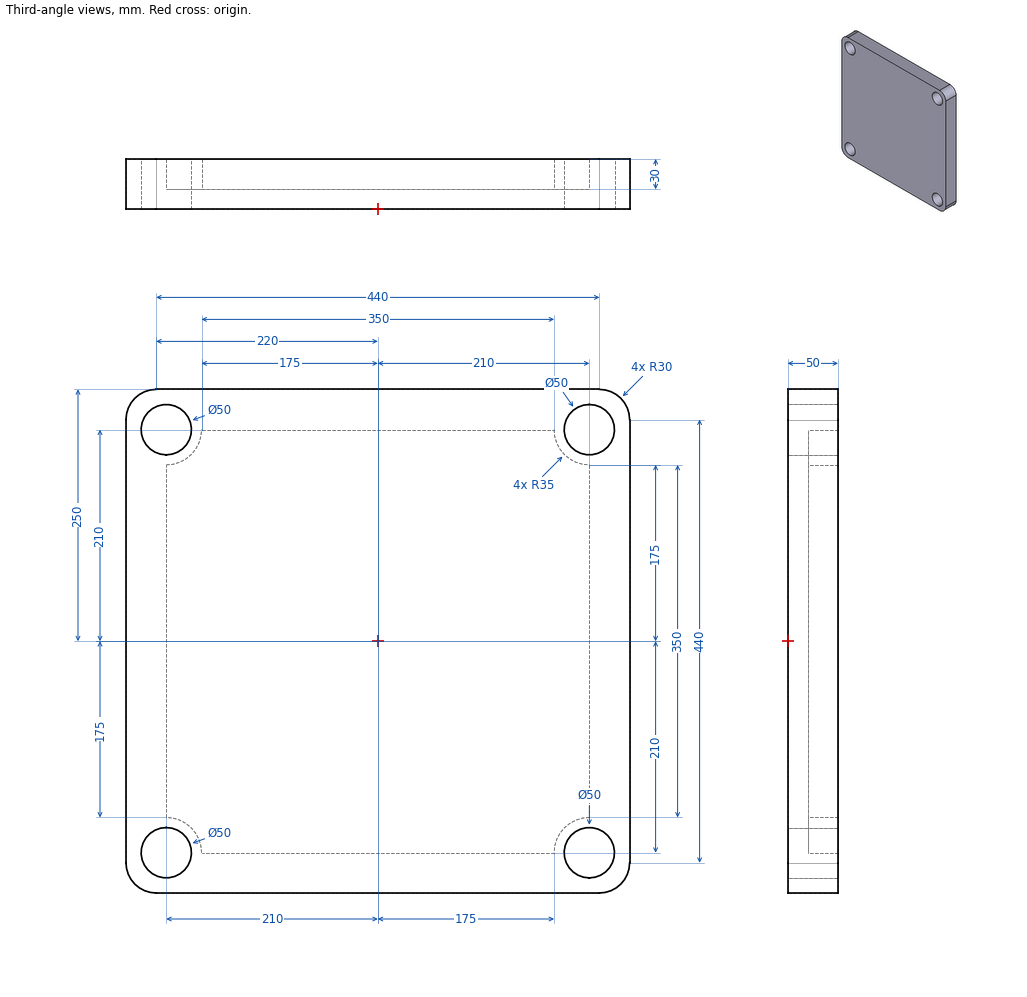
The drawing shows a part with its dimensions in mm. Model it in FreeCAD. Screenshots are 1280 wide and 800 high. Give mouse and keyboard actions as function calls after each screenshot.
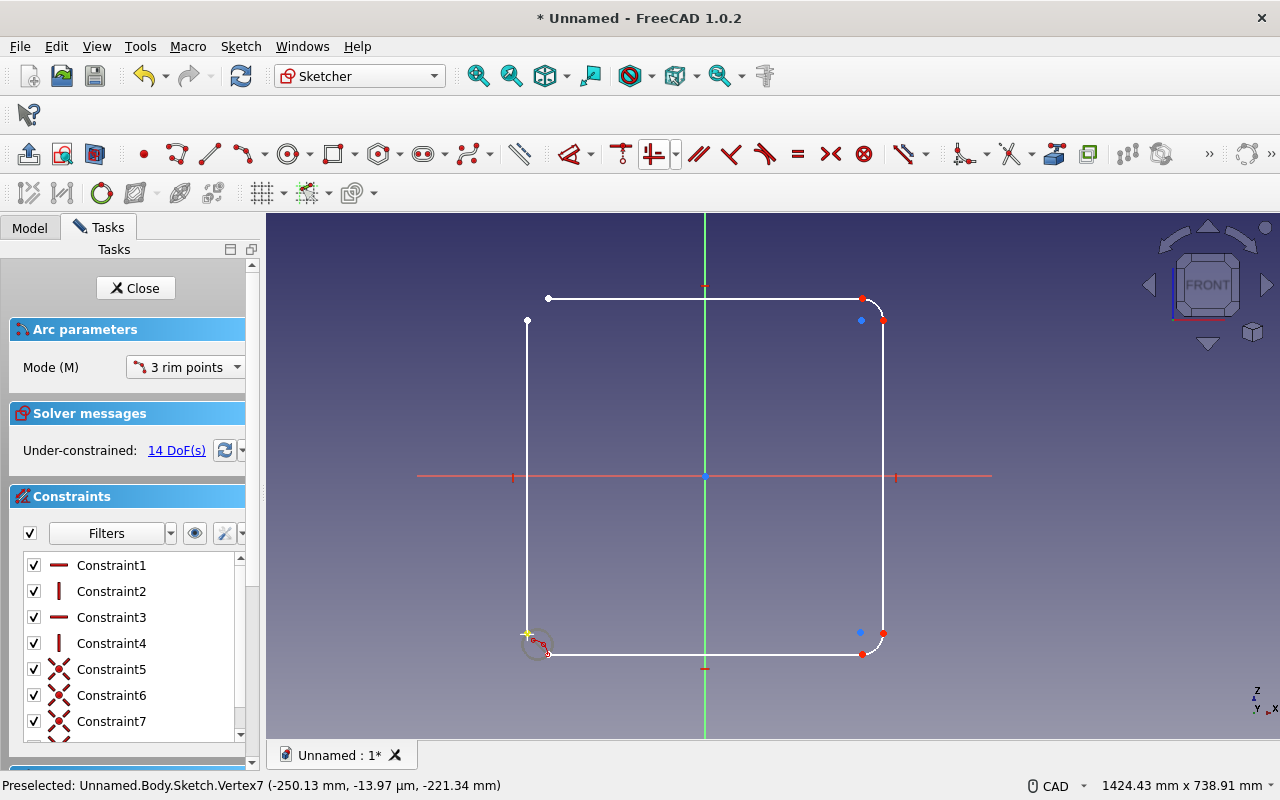
scroll(533, 648, up, 5)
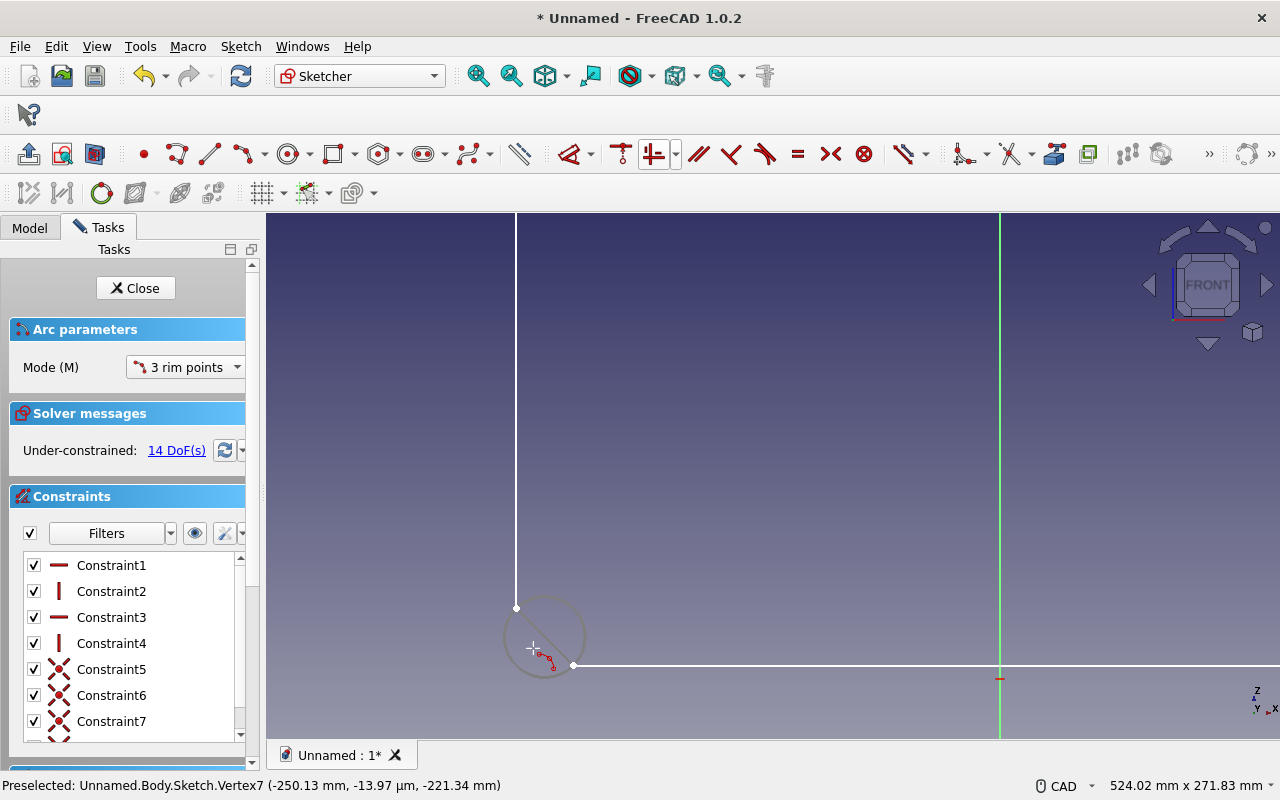
click(533, 647)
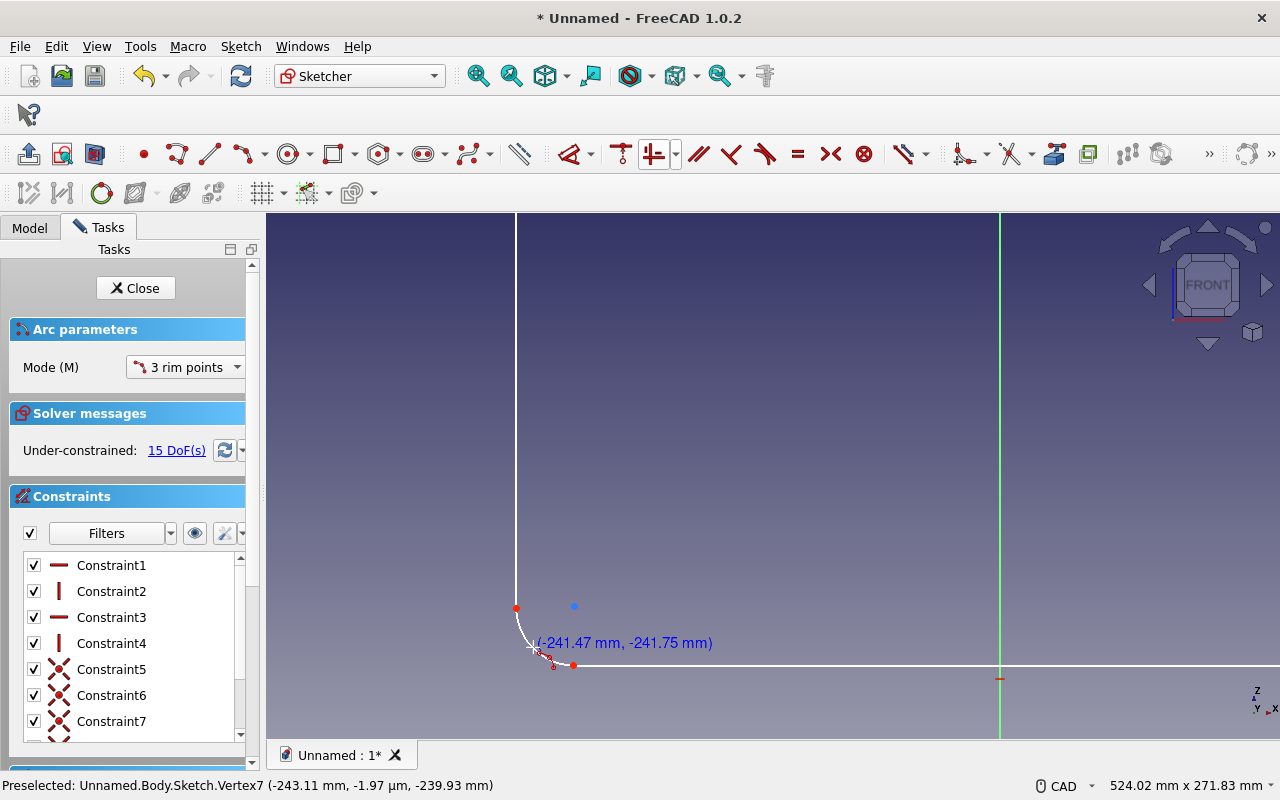
scroll(532, 648, down, 5)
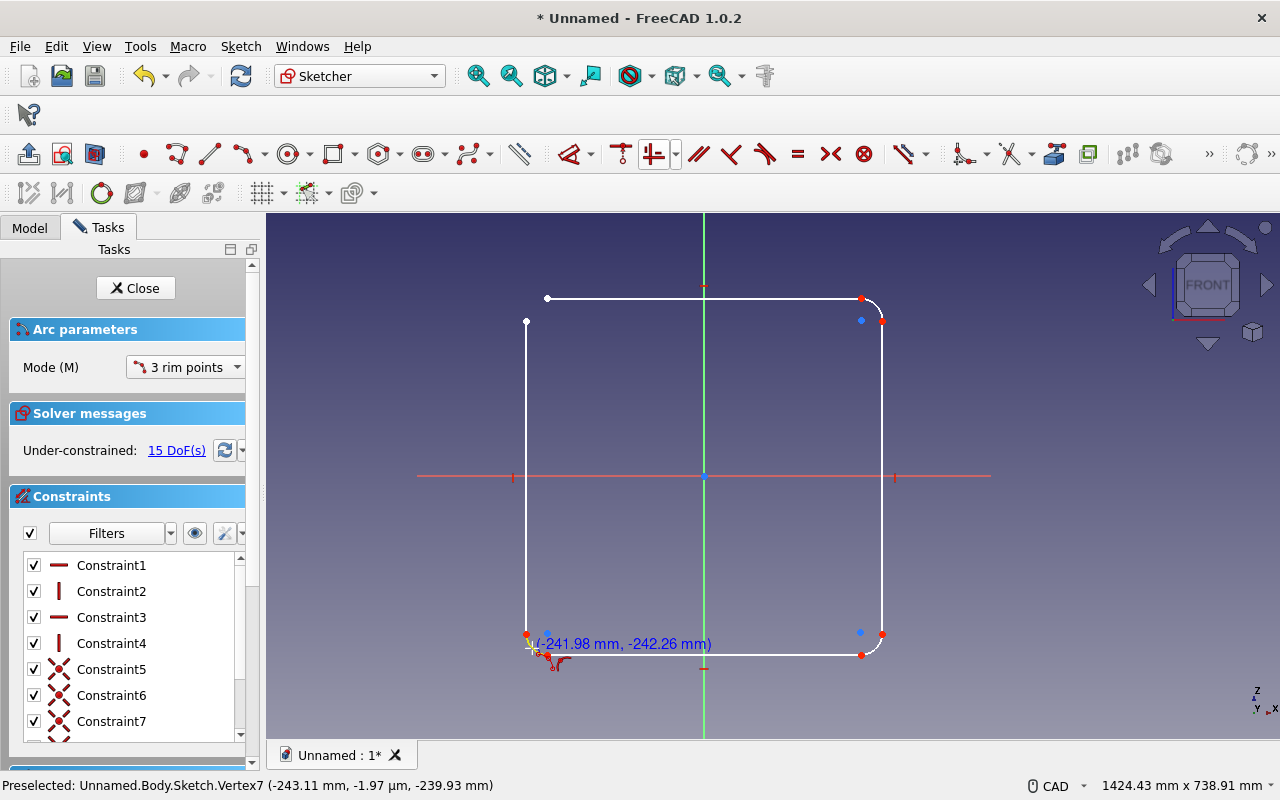
click(526, 321)
click(547, 299)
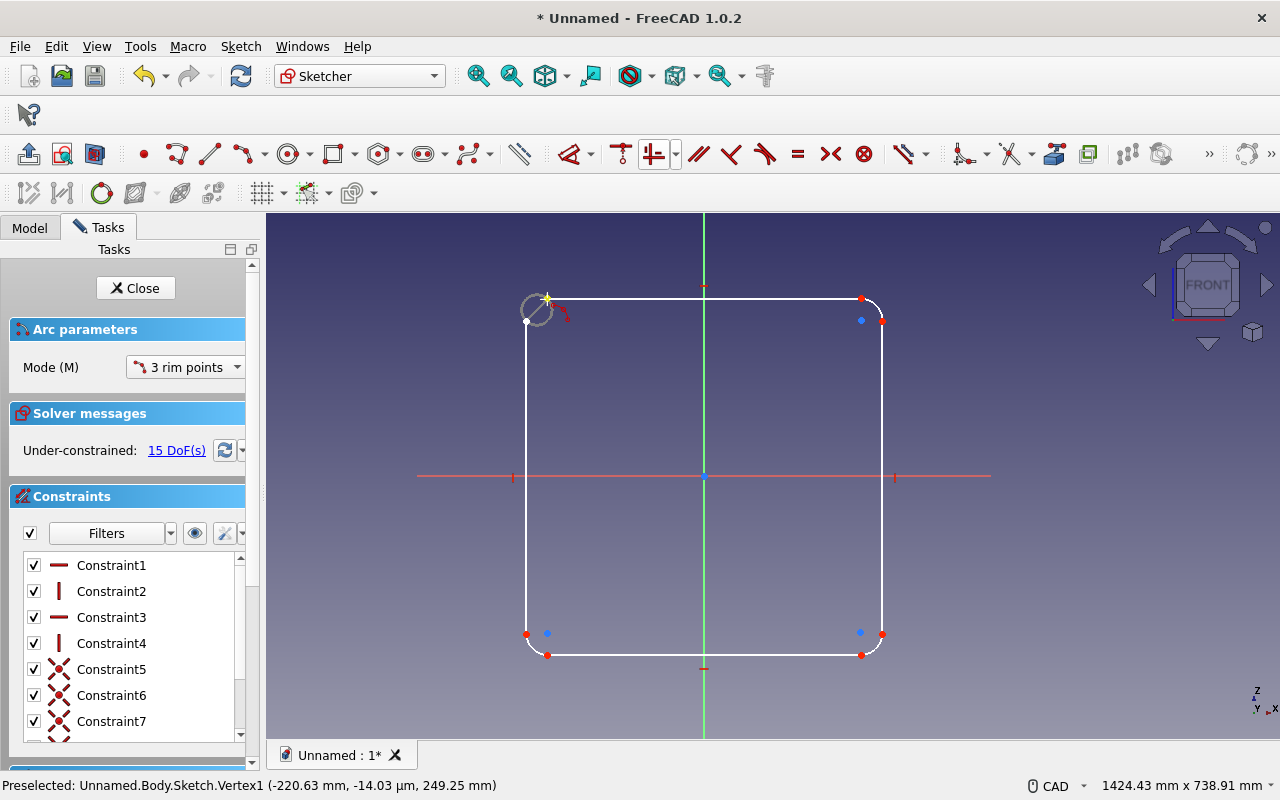
scroll(533, 305, up, 5)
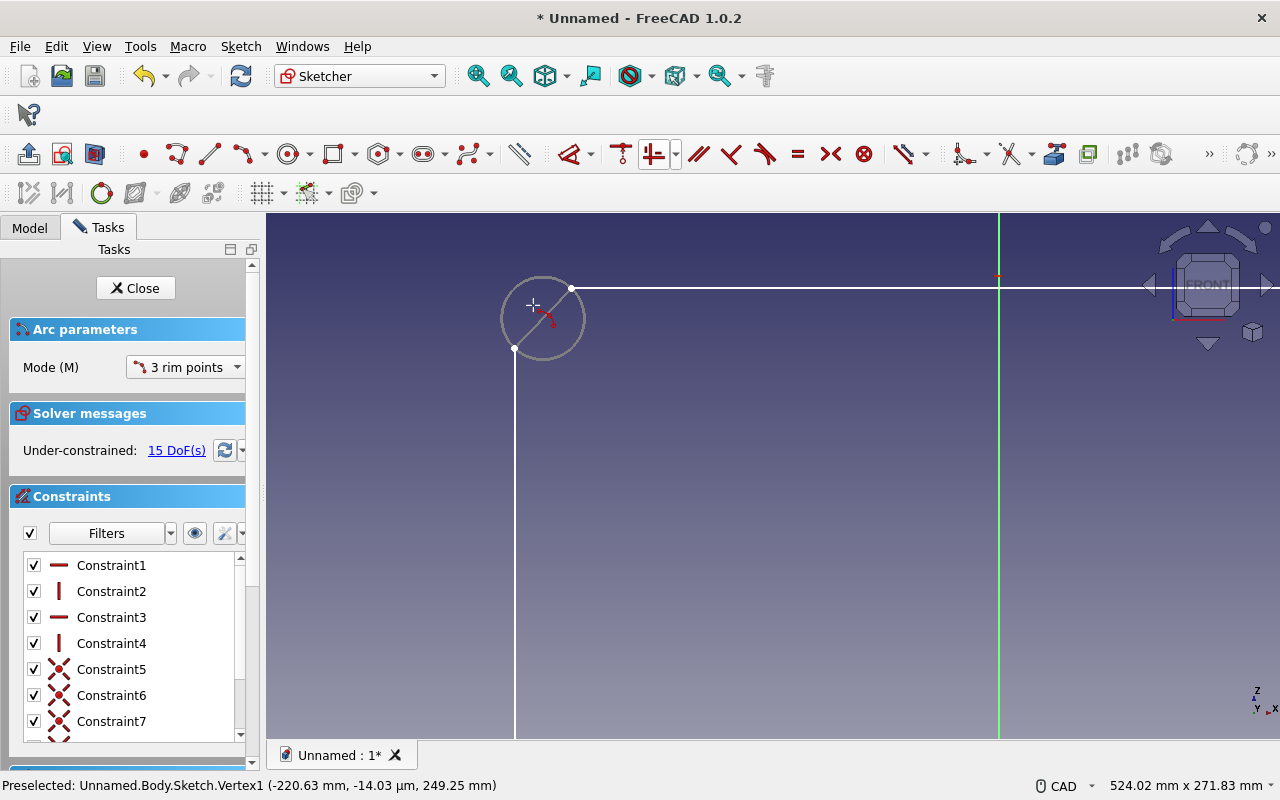
click(532, 304)
key(Escape)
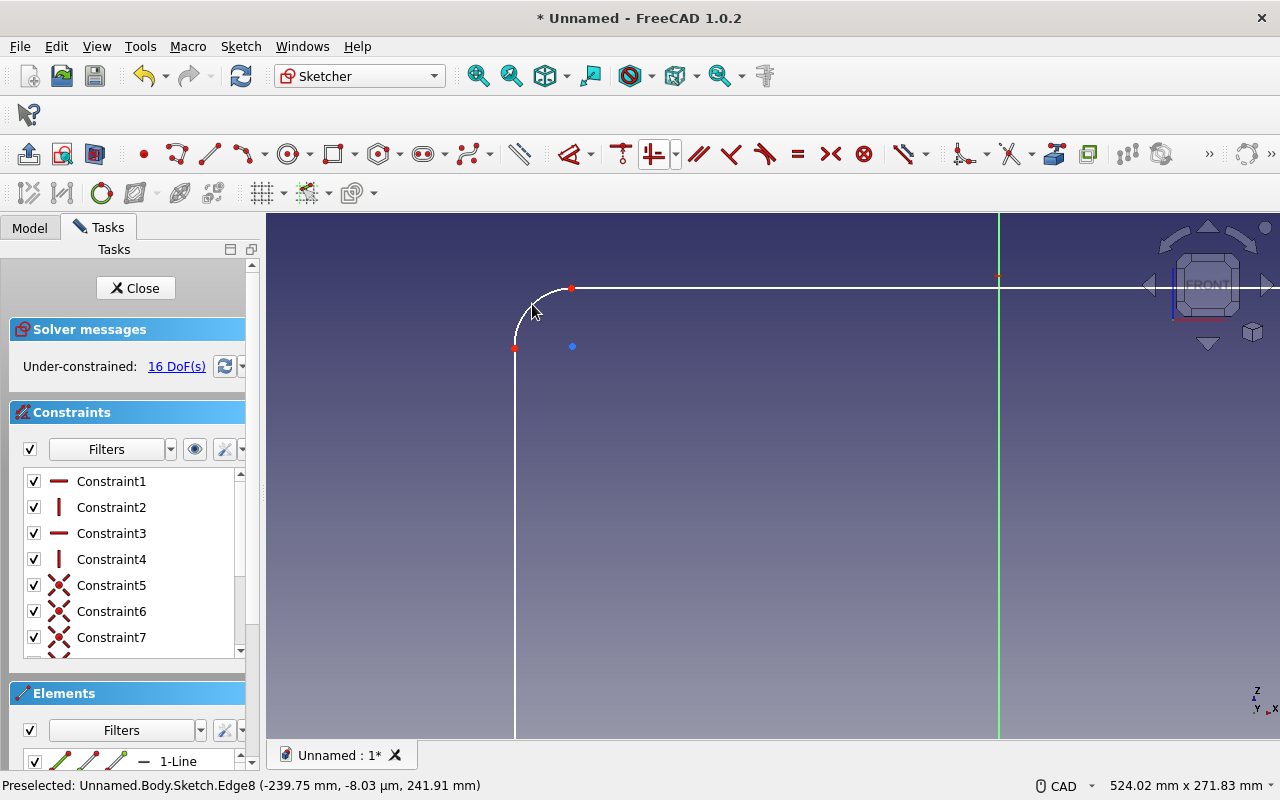
click(828, 288)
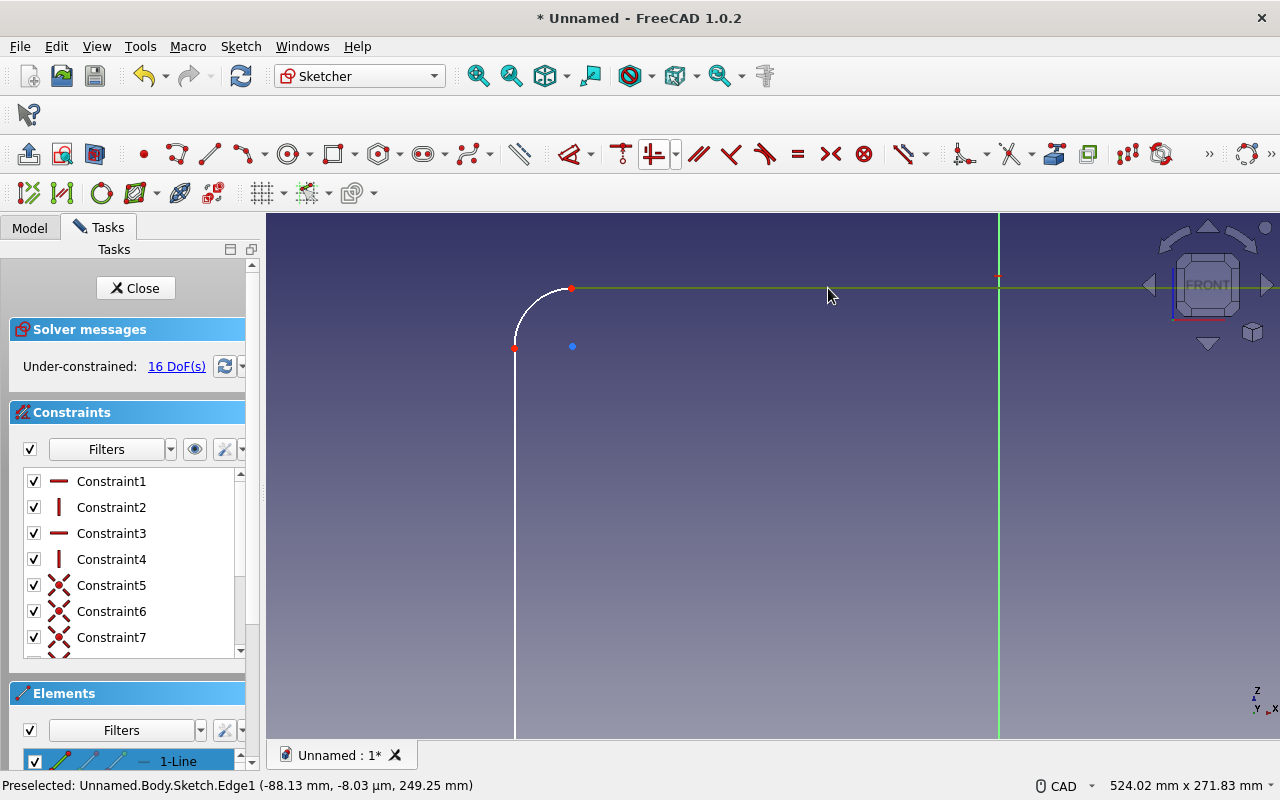
scroll(533, 304, down, 5)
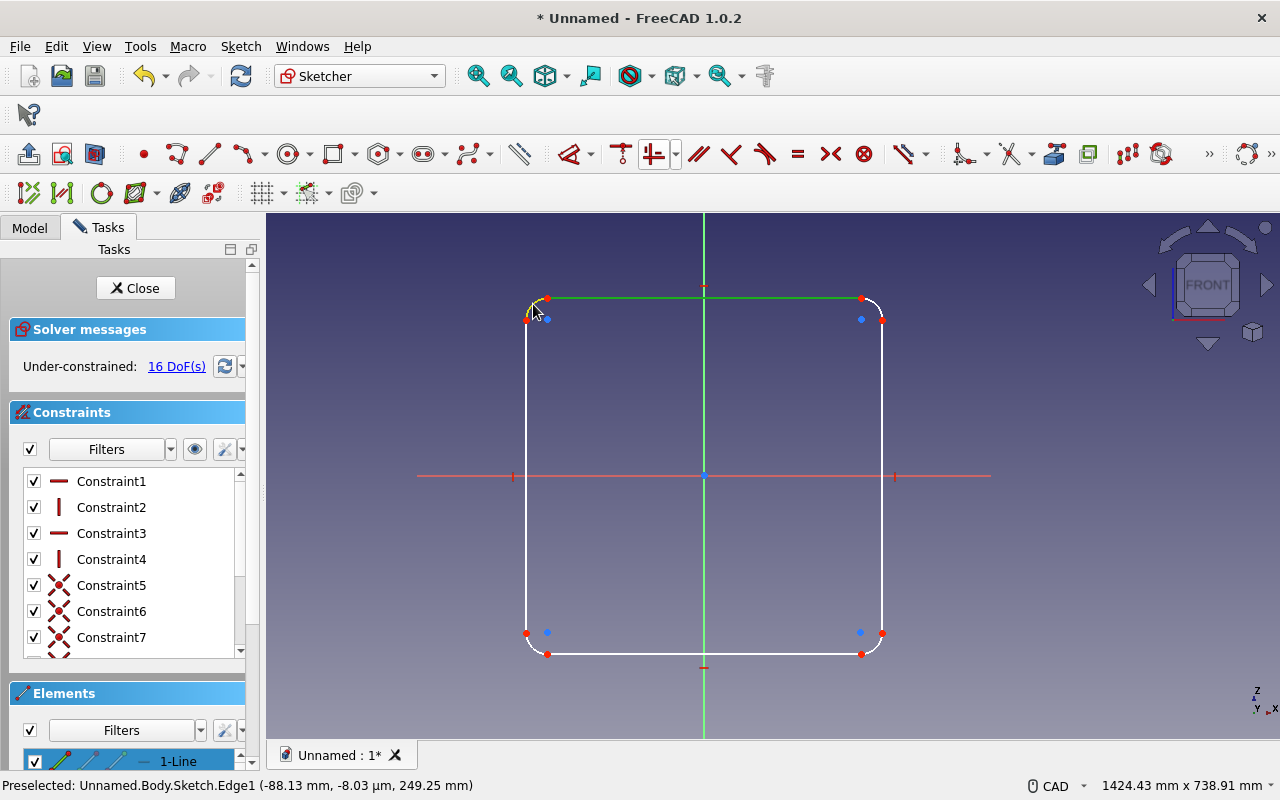
scroll(880, 311, up, 2)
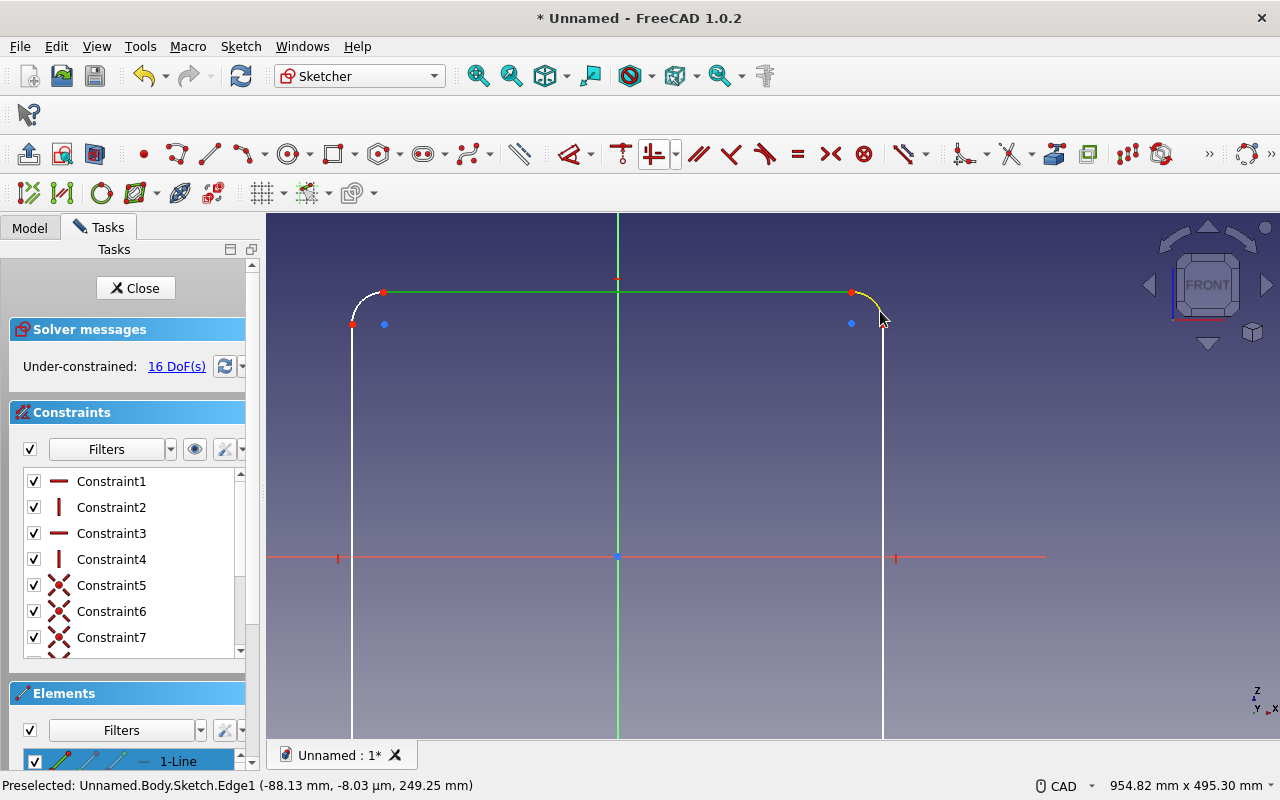
click(880, 310)